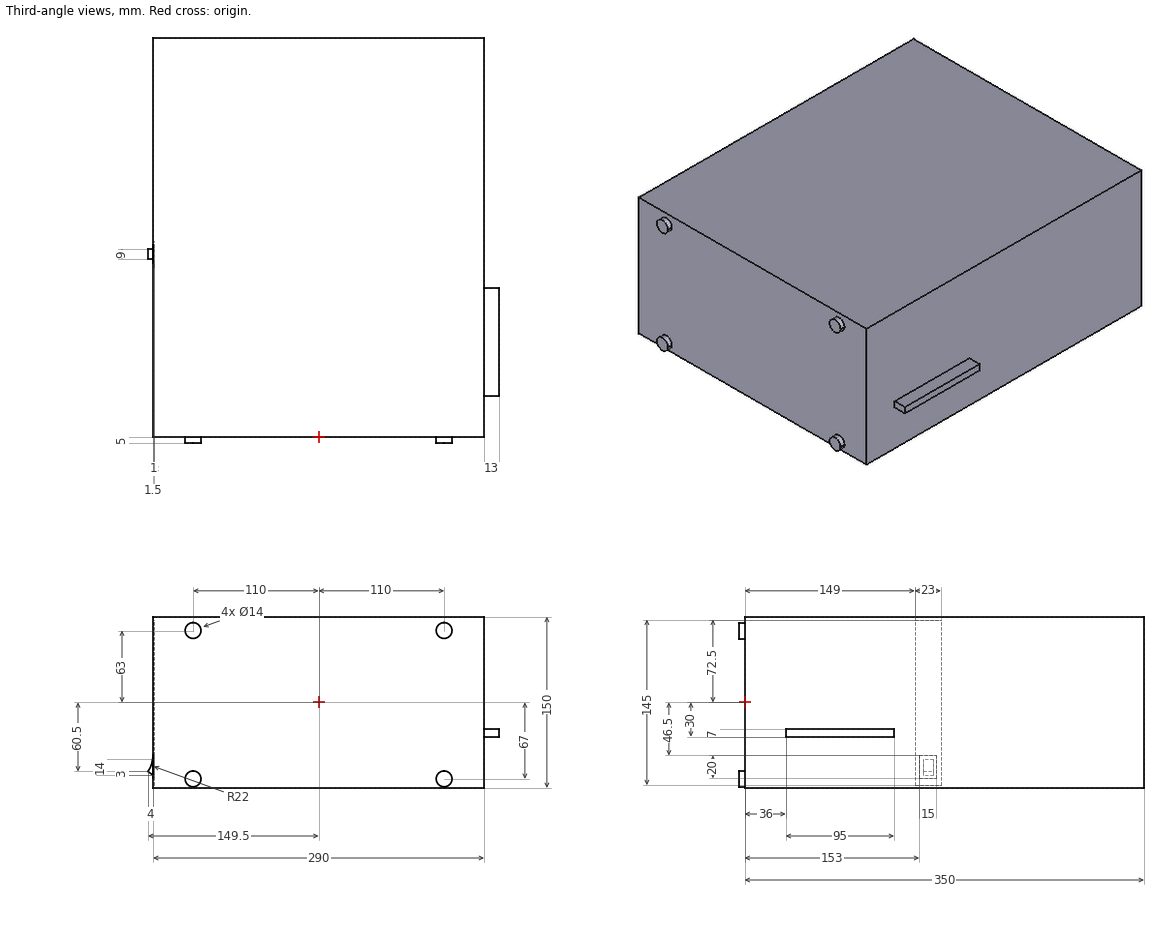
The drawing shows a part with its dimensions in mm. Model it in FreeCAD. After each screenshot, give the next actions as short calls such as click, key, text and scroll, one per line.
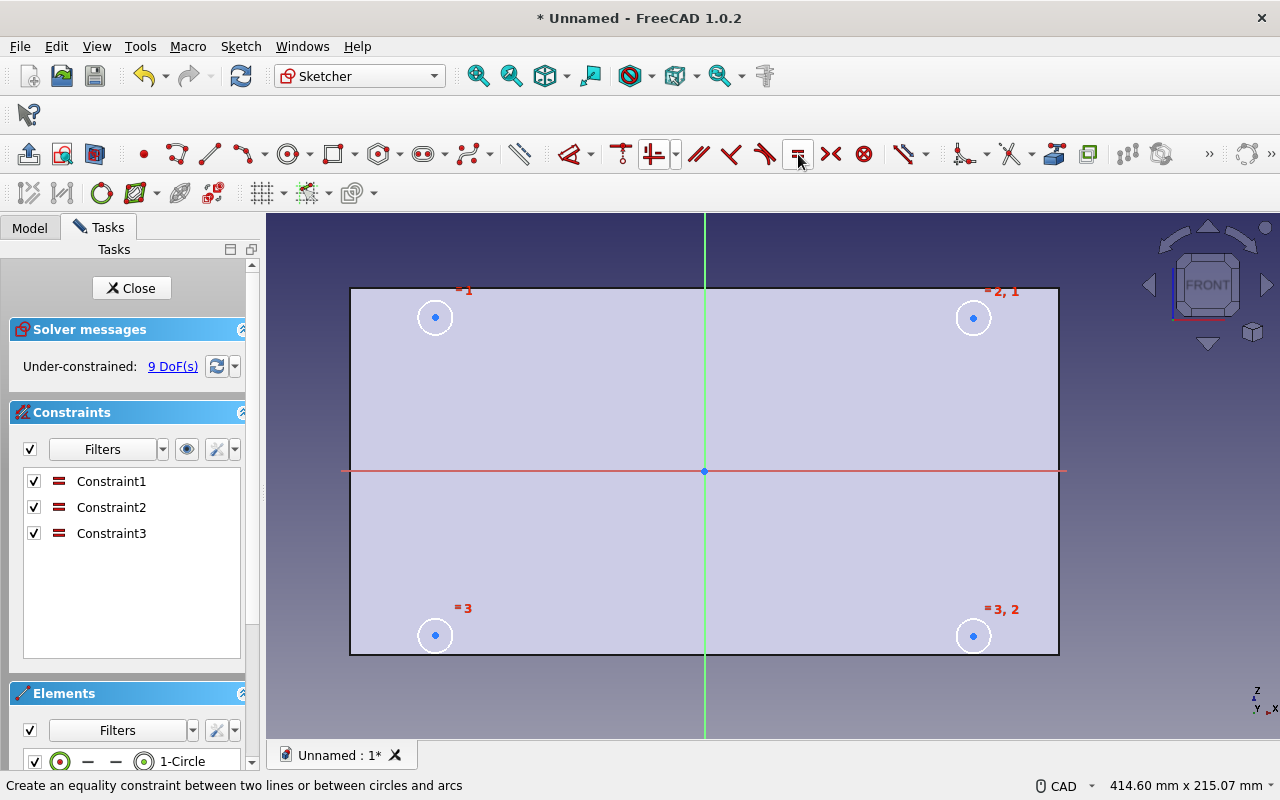
click(435, 318)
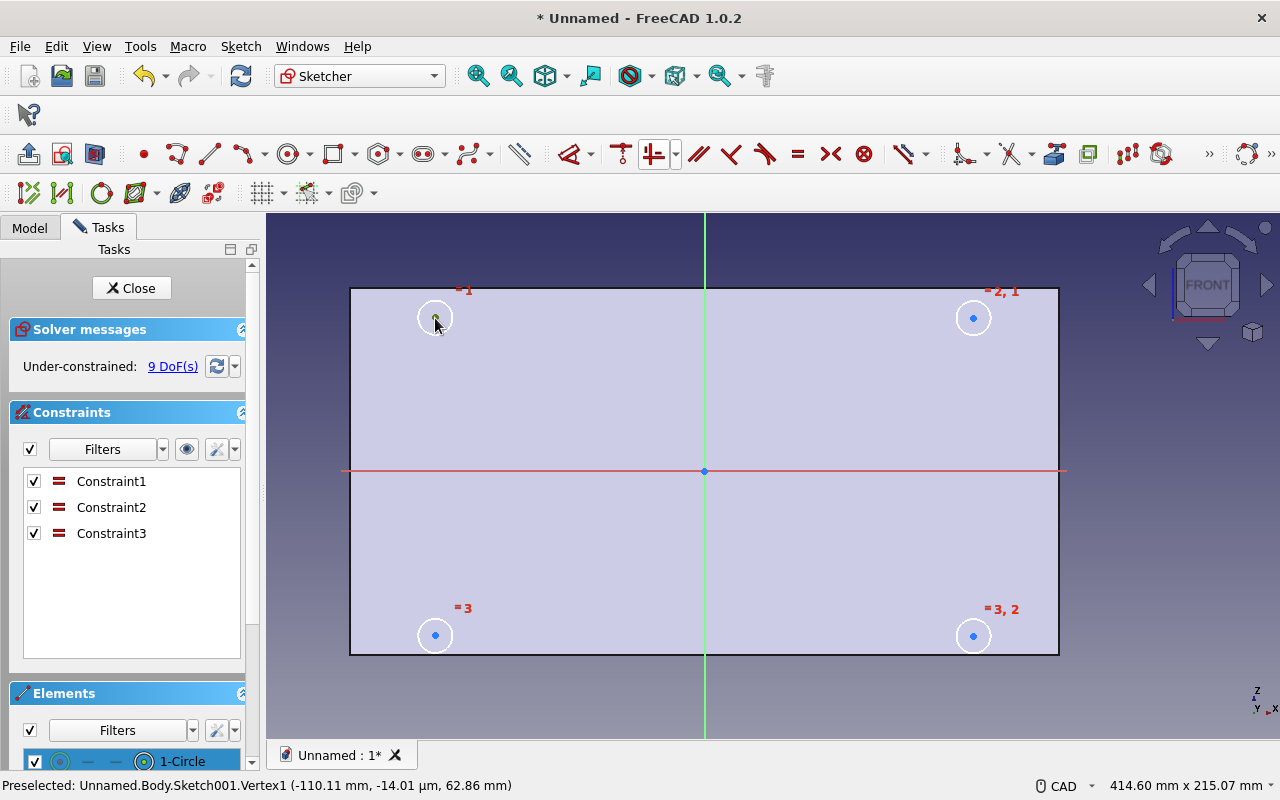
click(974, 318)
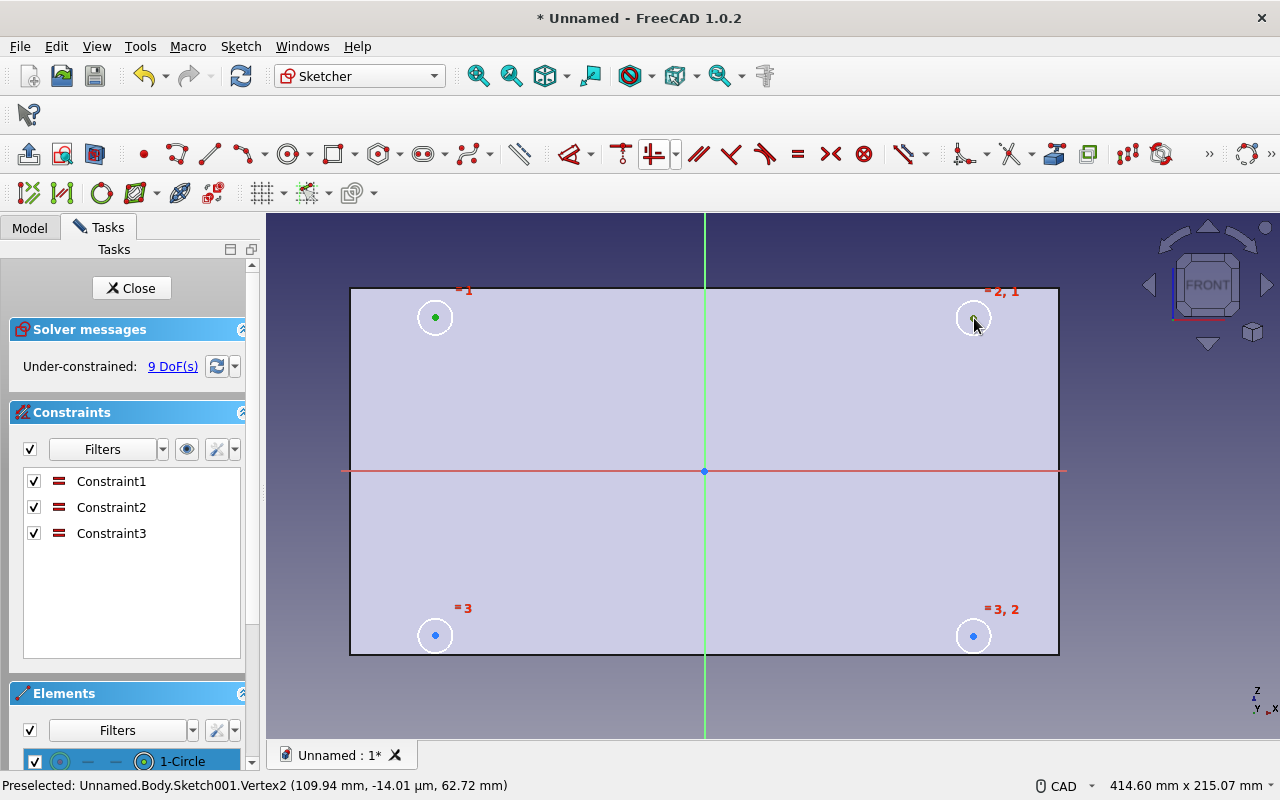
key(h)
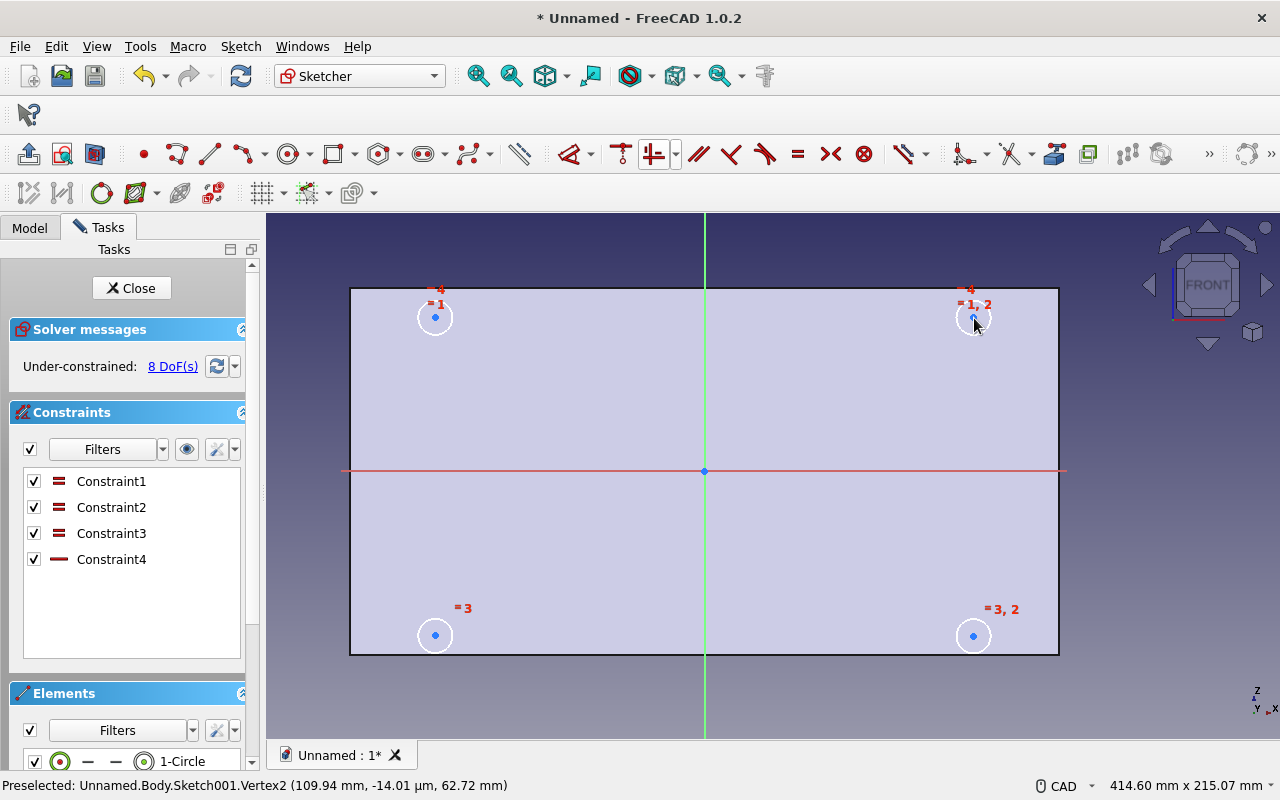
click(974, 318)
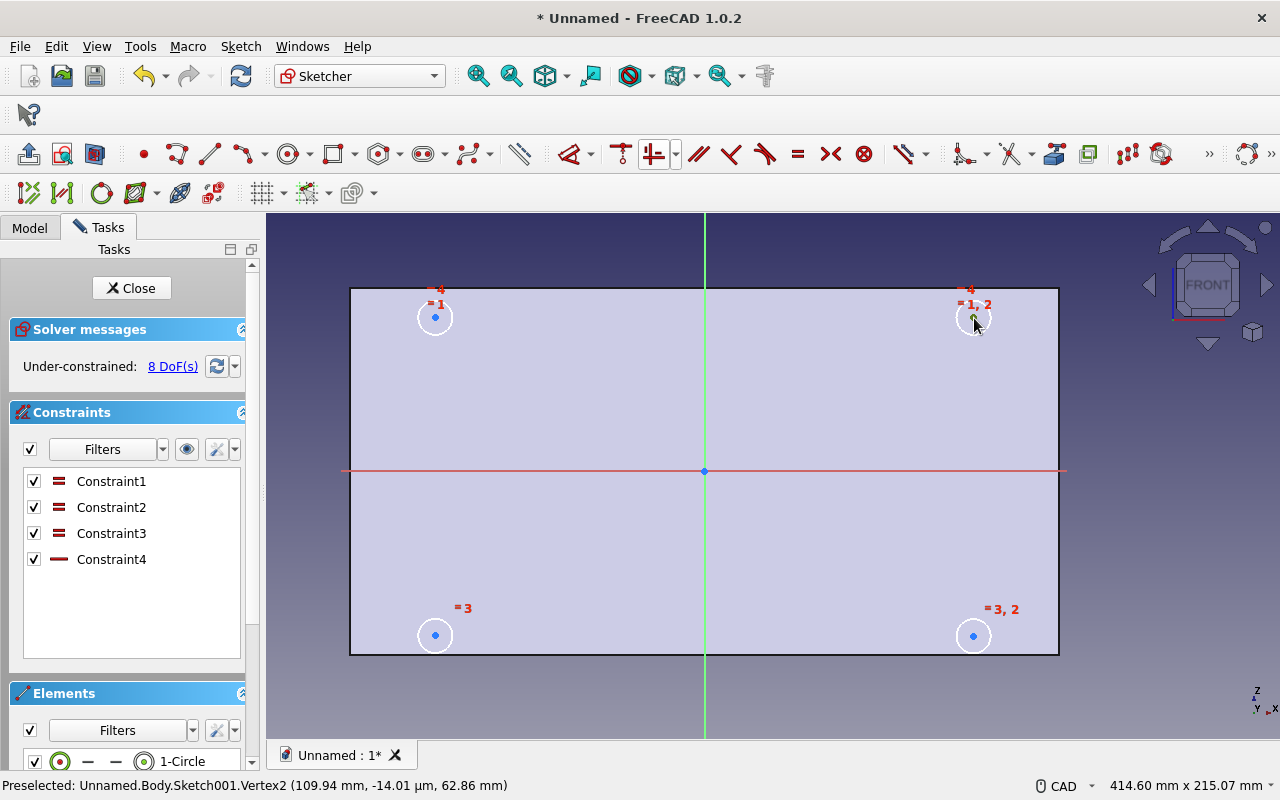
click(974, 636)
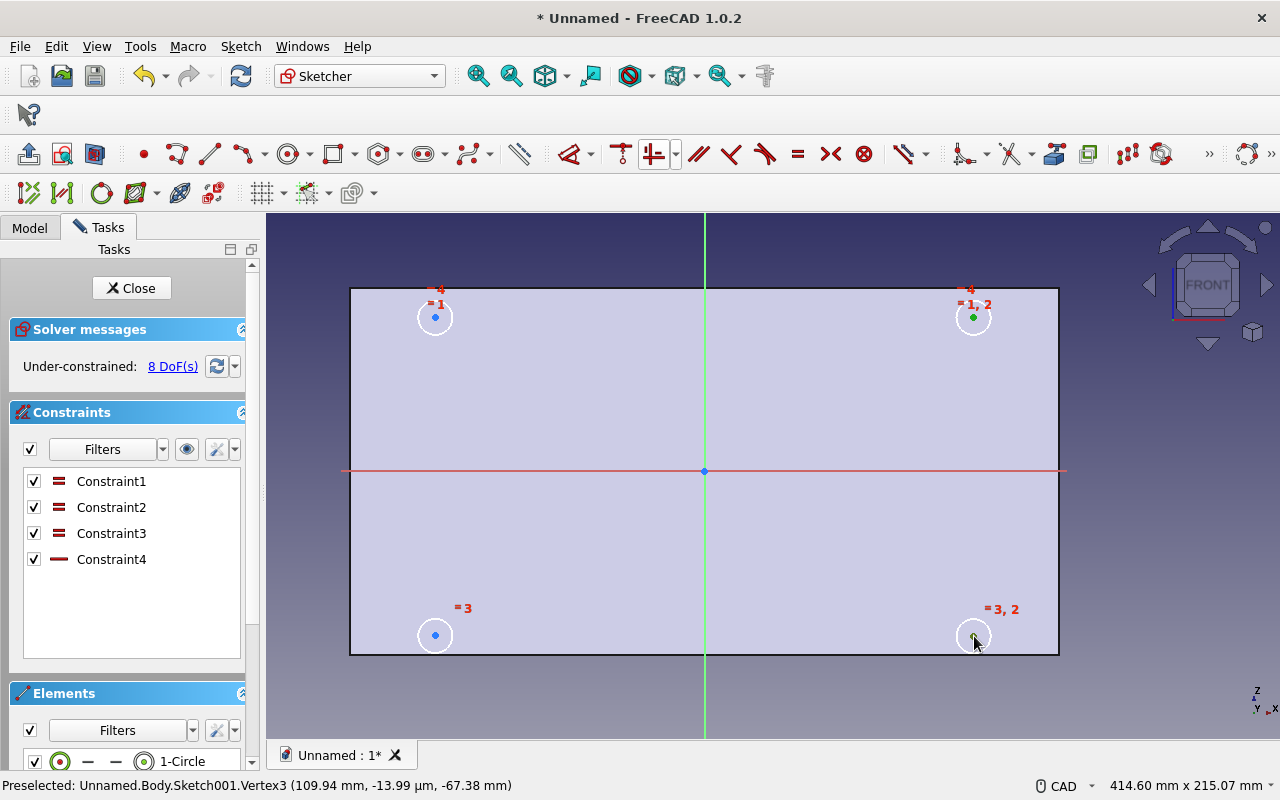
click(676, 154)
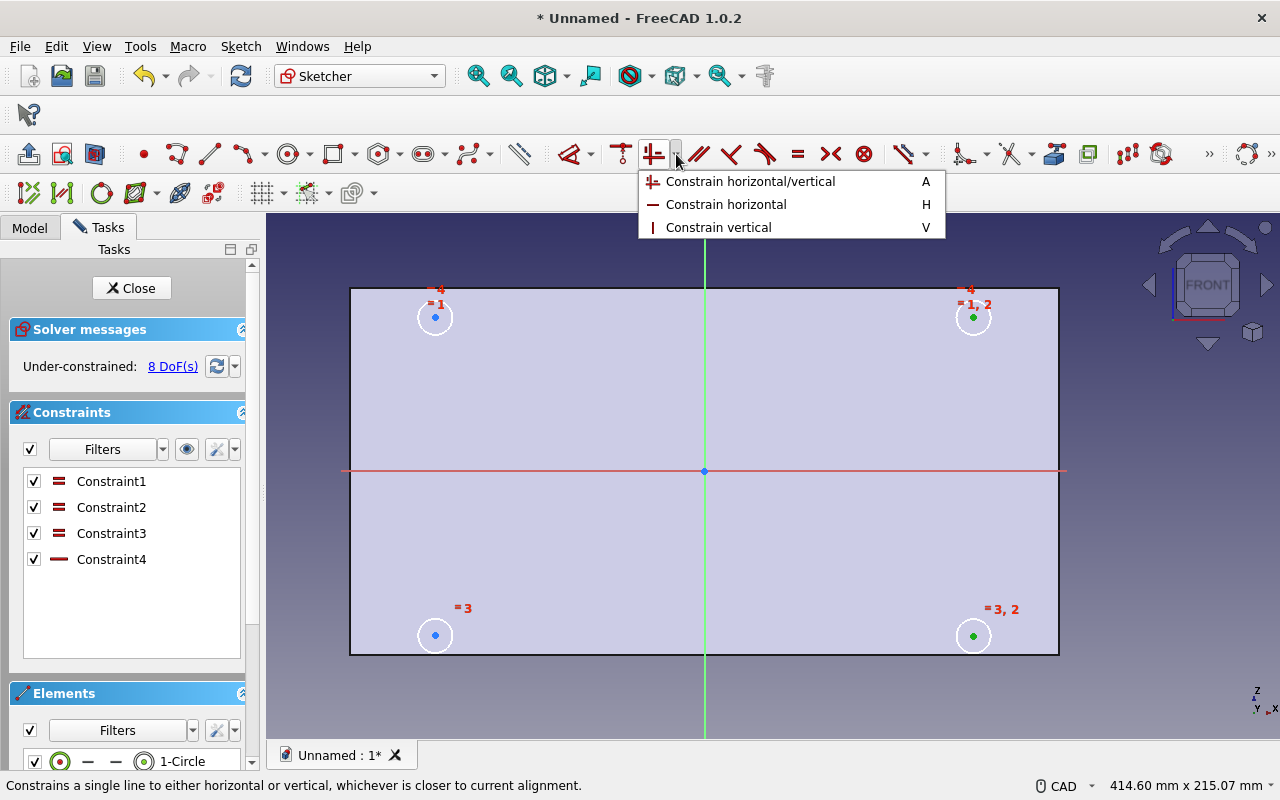
click(792, 228)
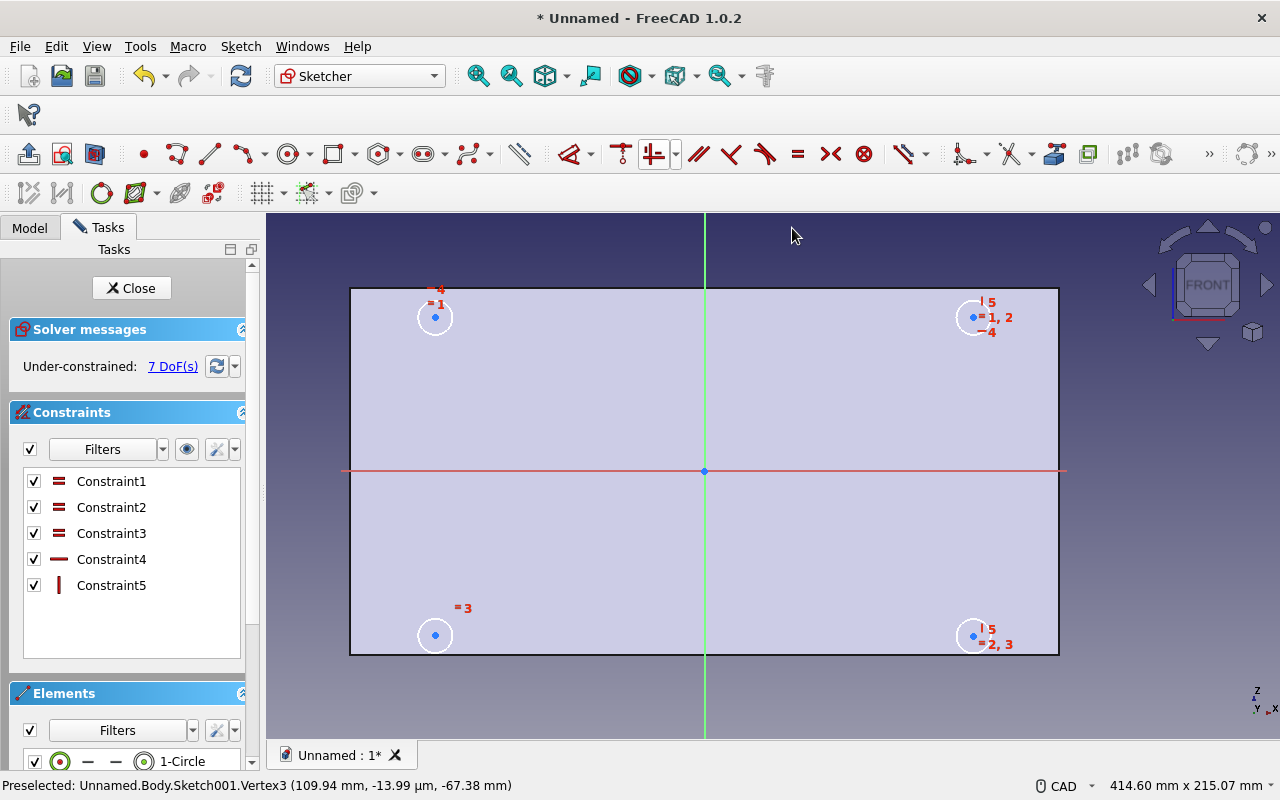
click(435, 318)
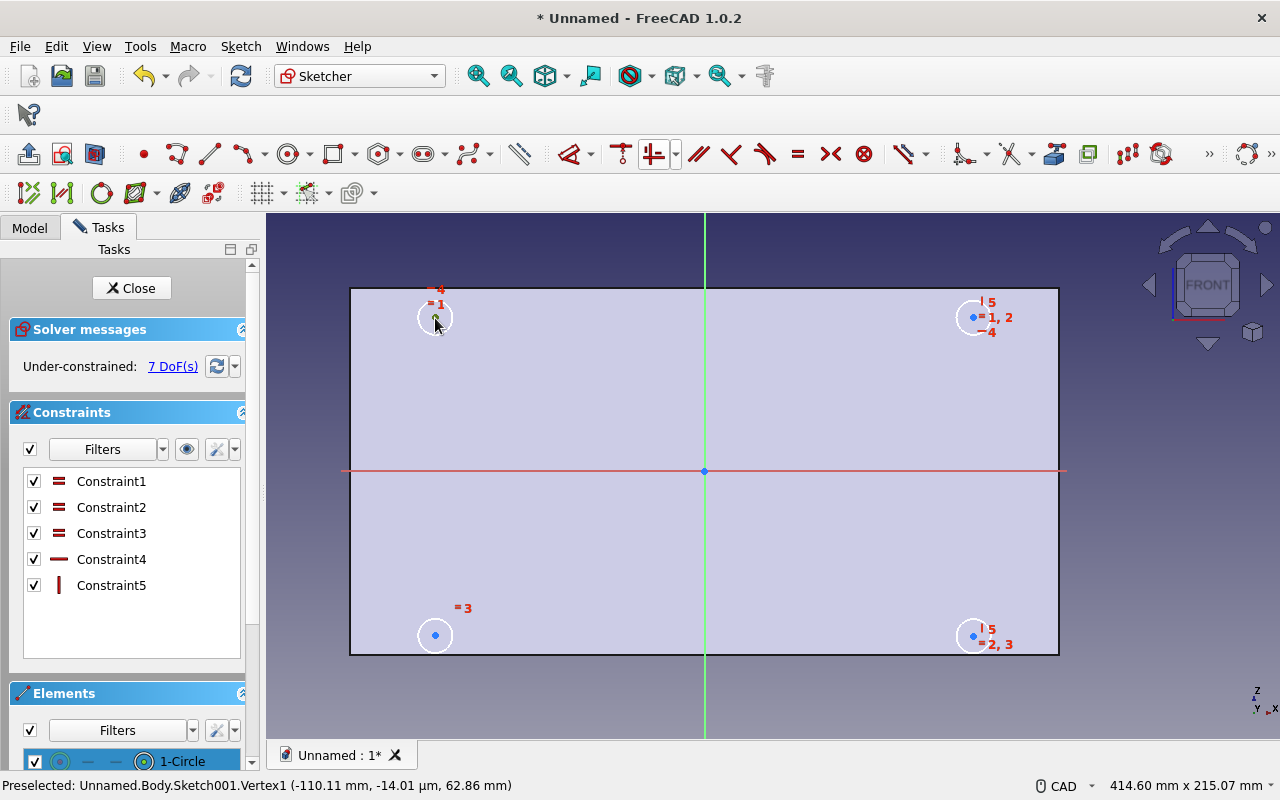
click(435, 636)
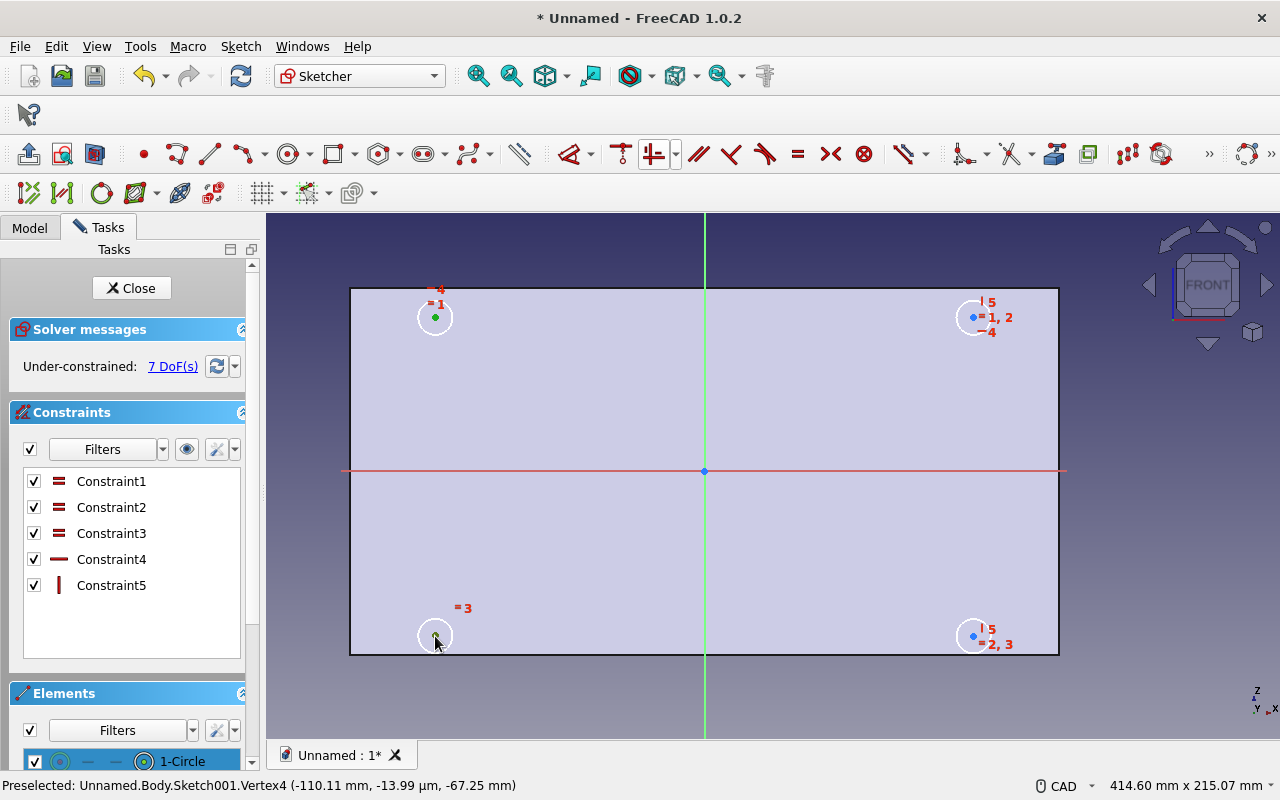
key(v)